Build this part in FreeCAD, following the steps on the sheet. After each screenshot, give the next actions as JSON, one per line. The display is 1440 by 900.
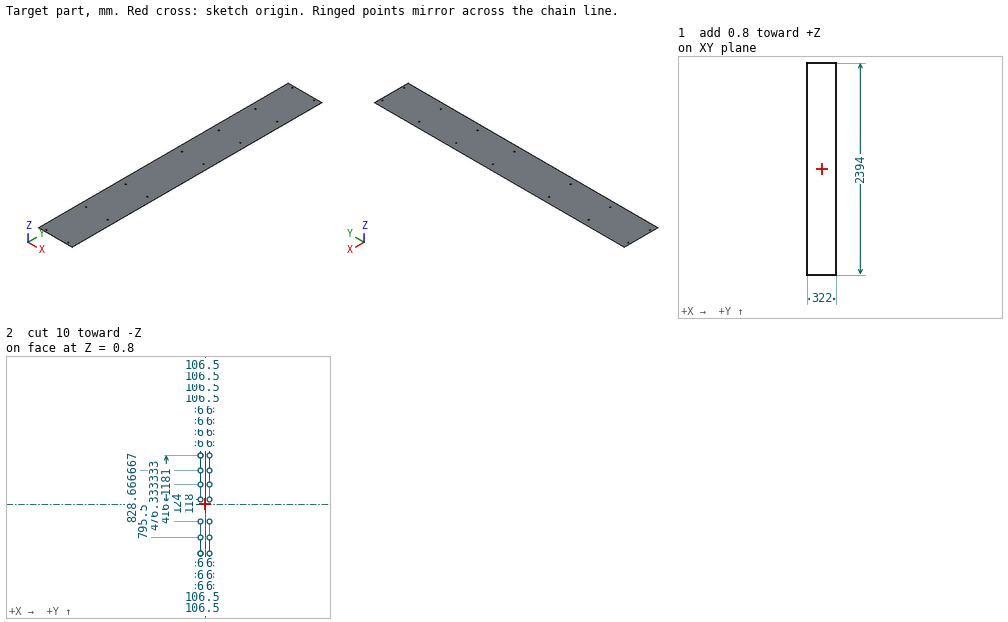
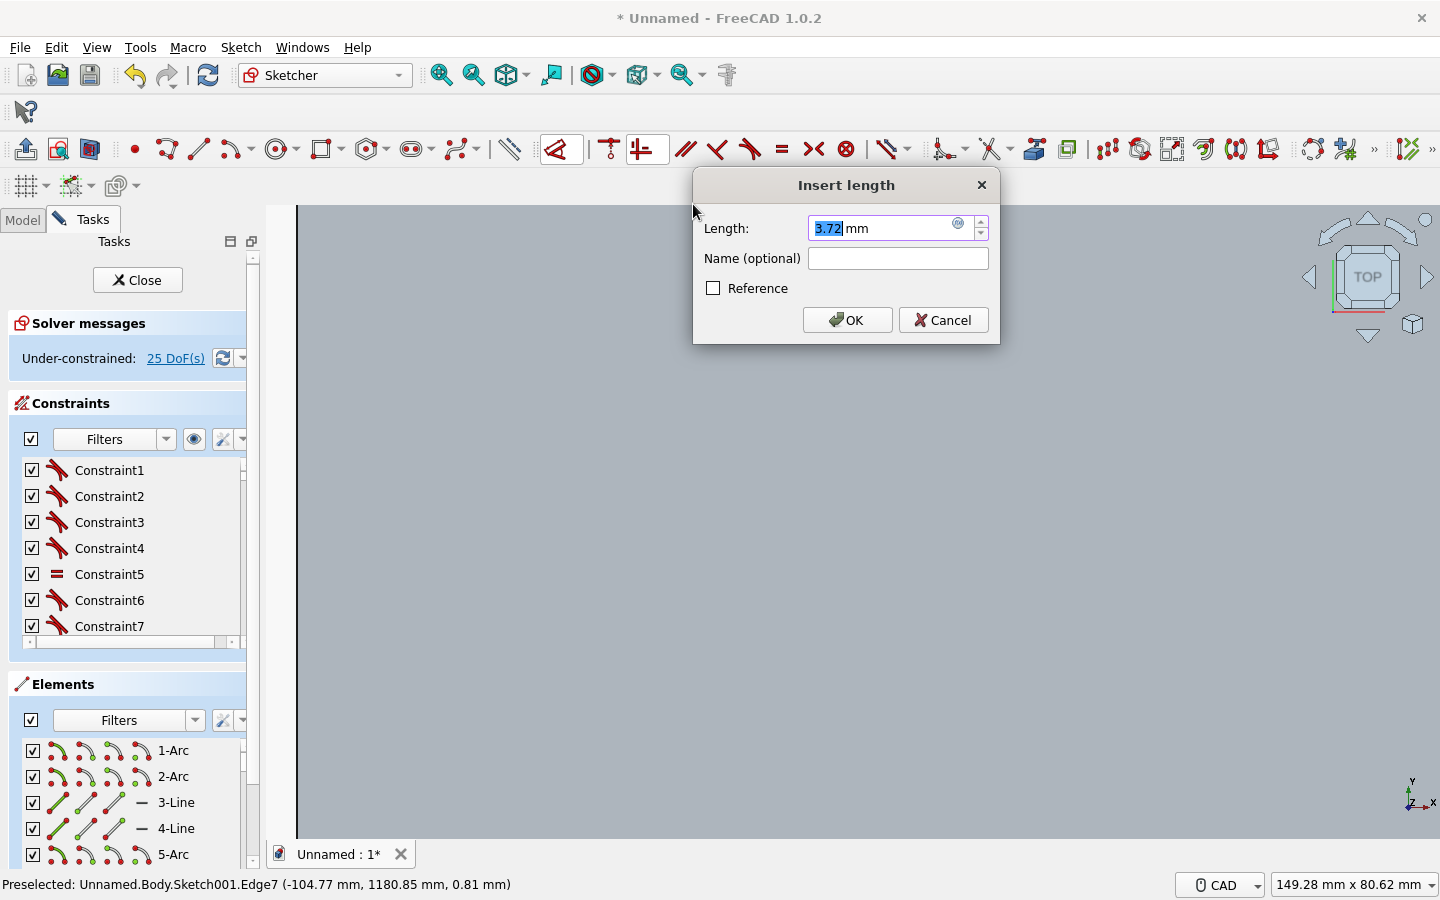
{"action": "type", "text": "6"}
{"action": "key", "text": "Return"}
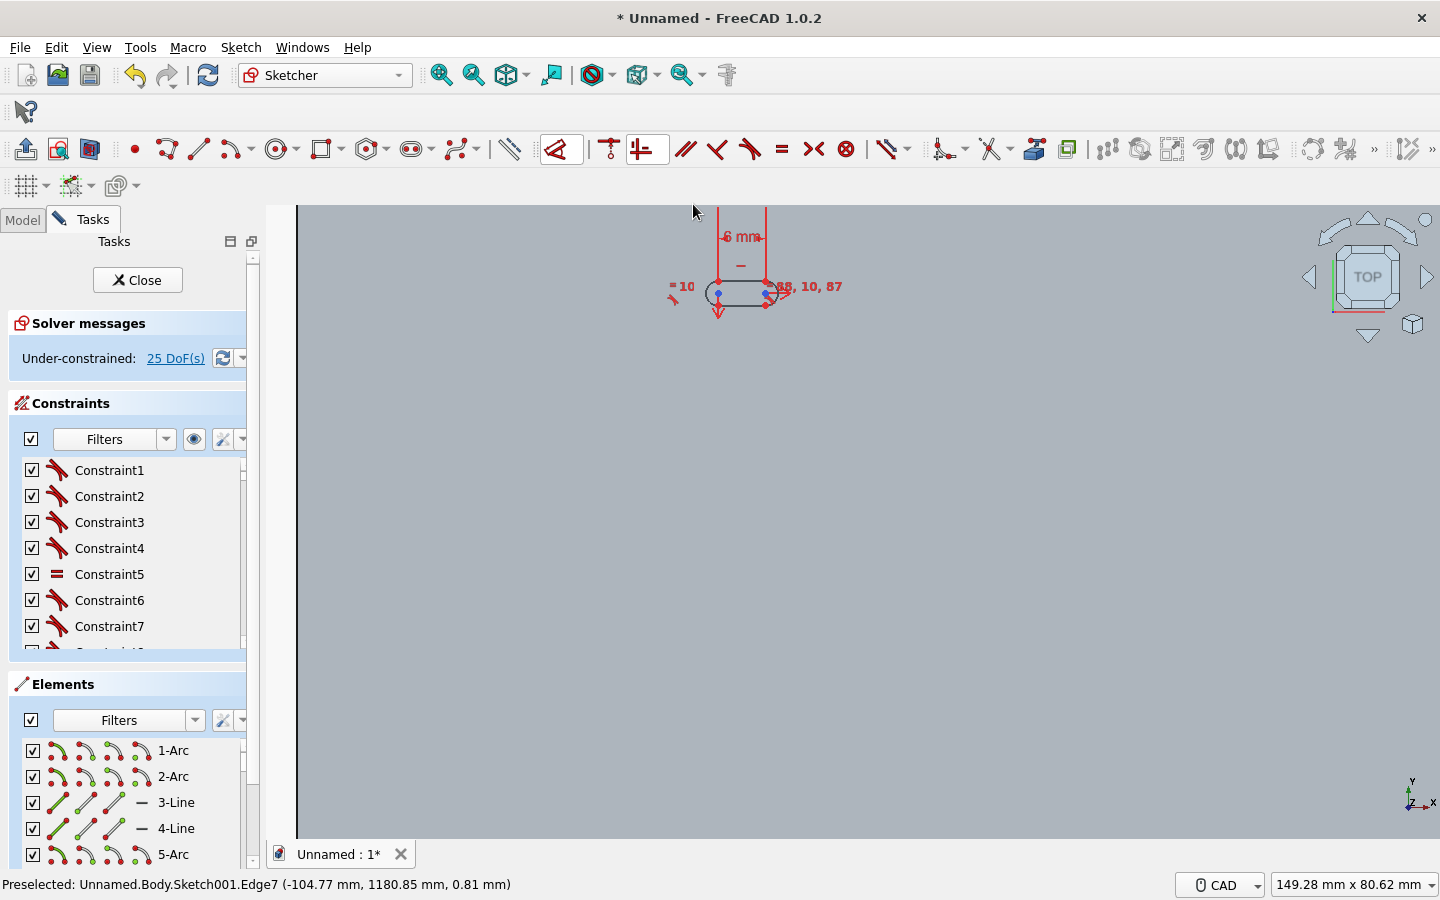
{"action": "scroll", "coordinate": [763, 268], "scroll_direction": "down", "scroll_amount": 18}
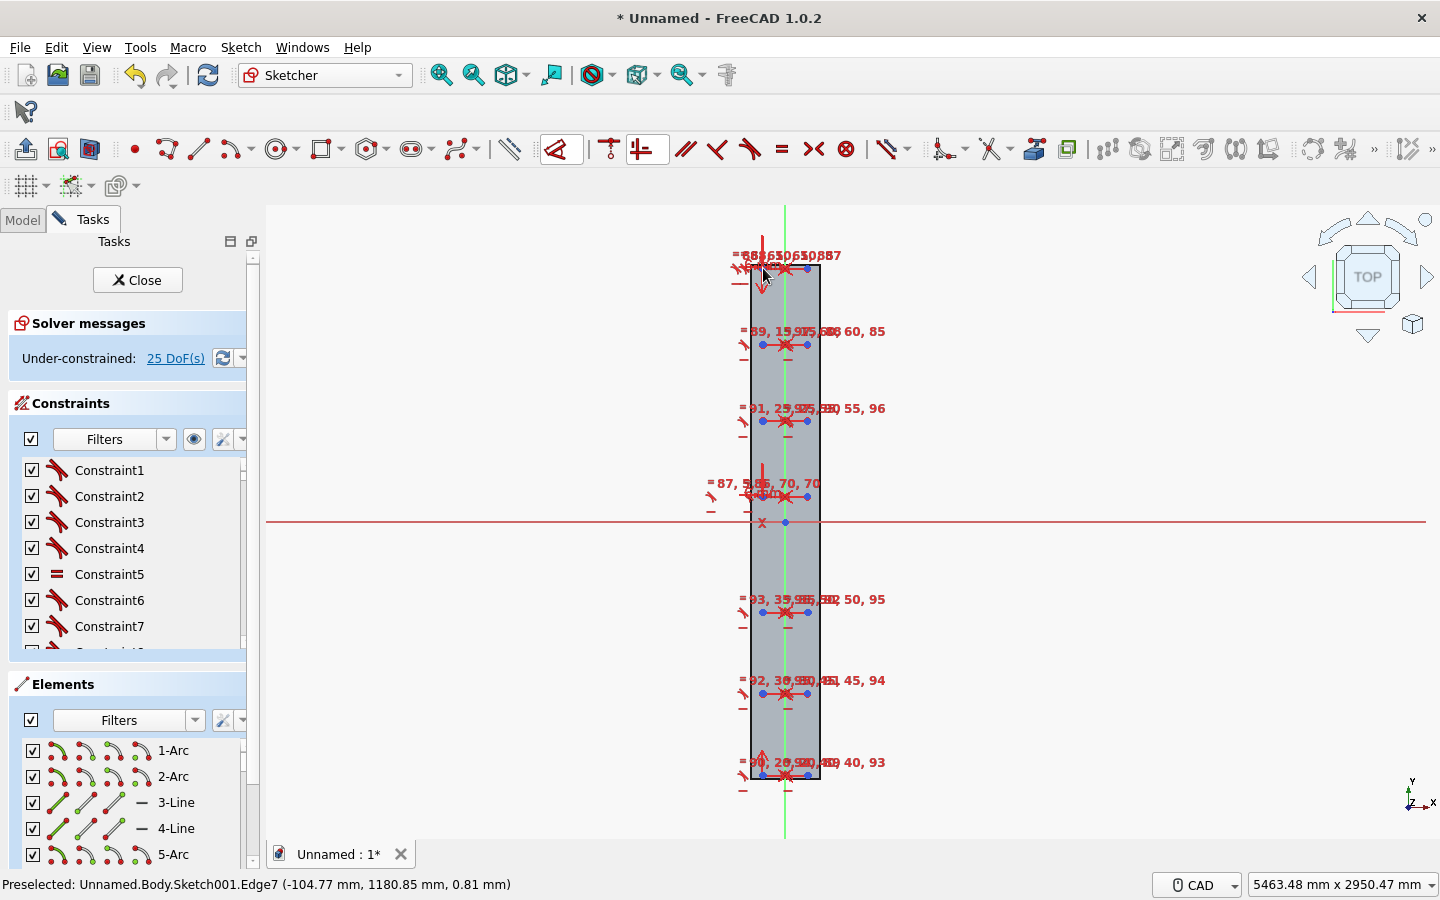
{"action": "scroll", "coordinate": [763, 345], "scroll_direction": "up", "scroll_amount": 18}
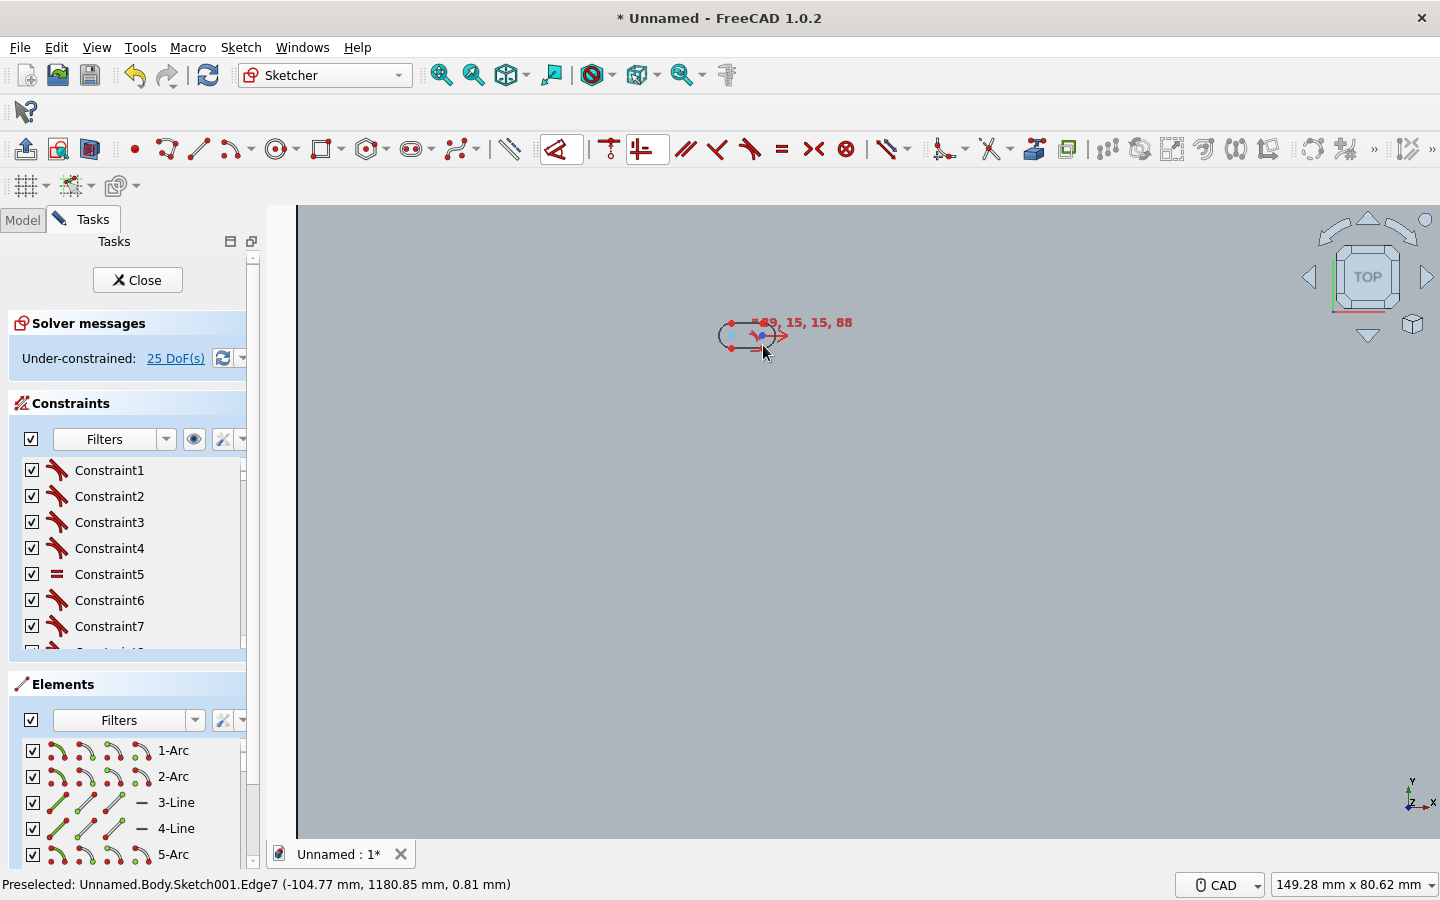
{"action": "left_click", "coordinate": [741, 323]}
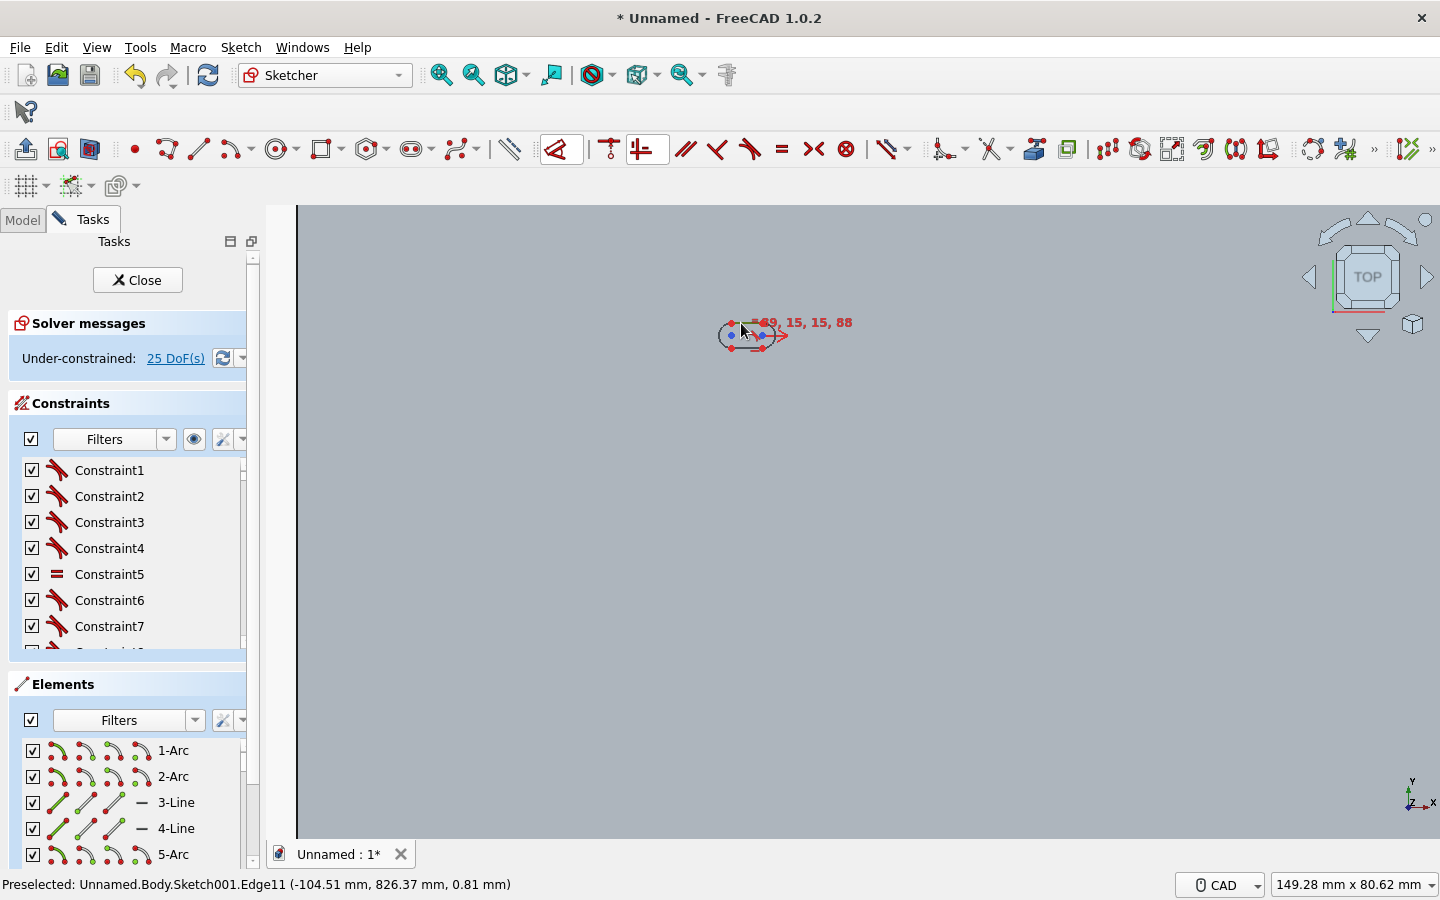
{"action": "key", "text": "l"}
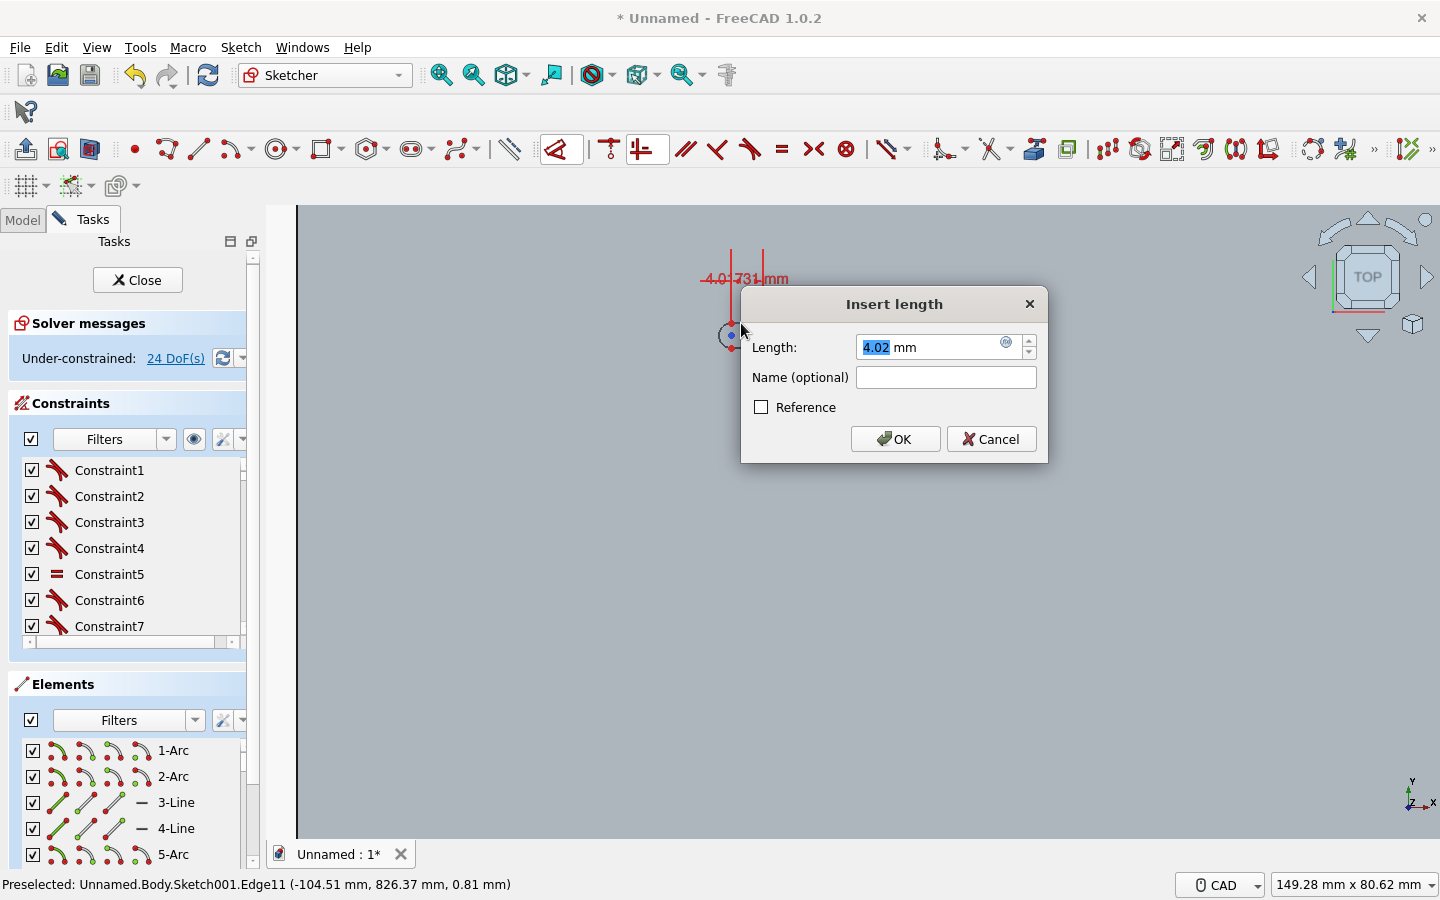
{"action": "type", "text": "6"}
{"action": "key", "text": "Return"}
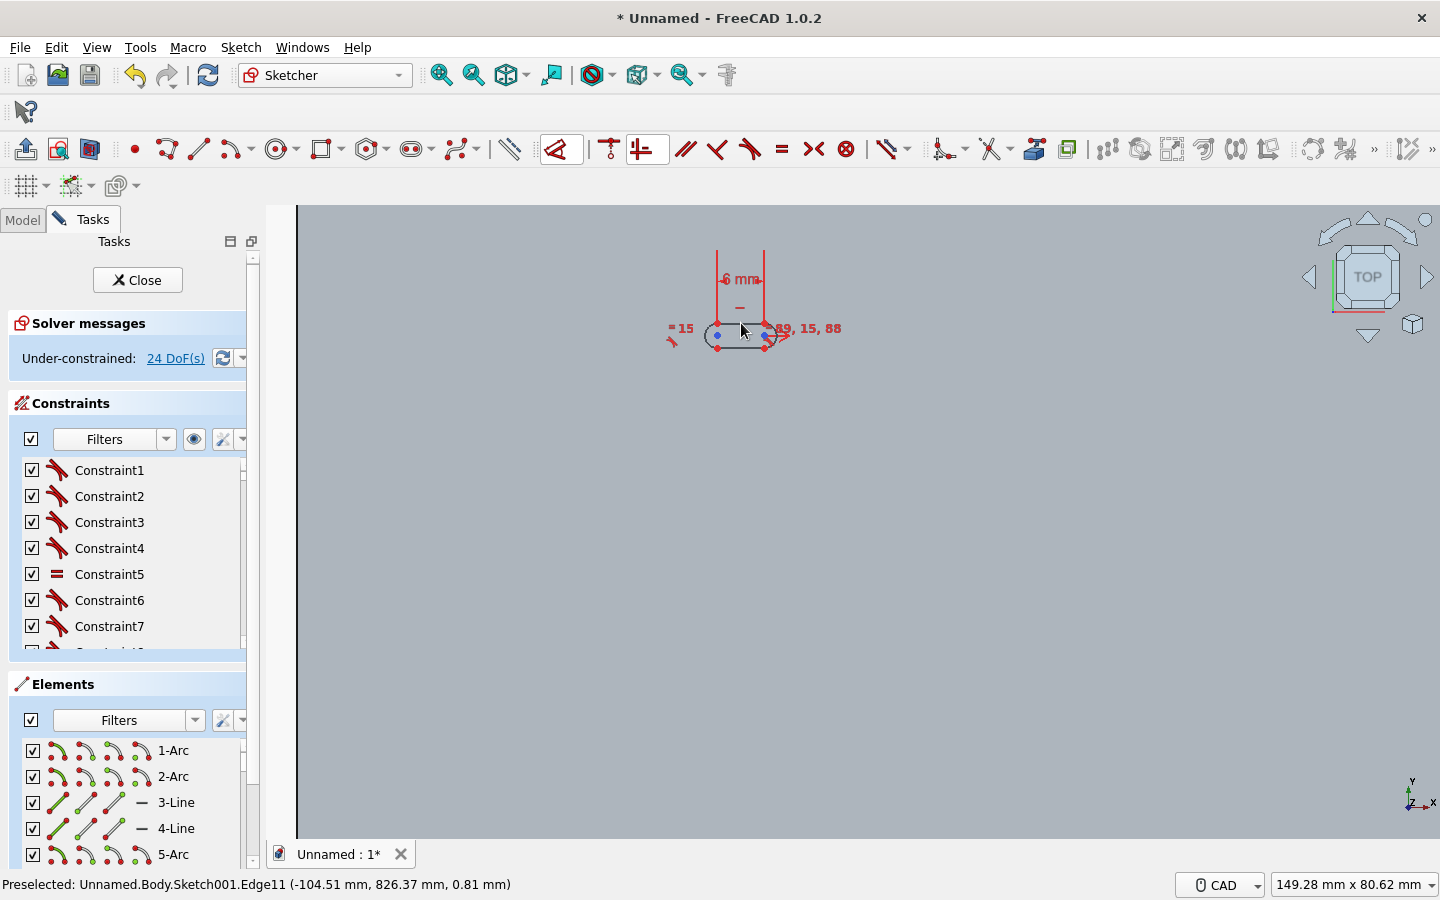
{"action": "scroll", "coordinate": [763, 345], "scroll_direction": "down", "scroll_amount": 18}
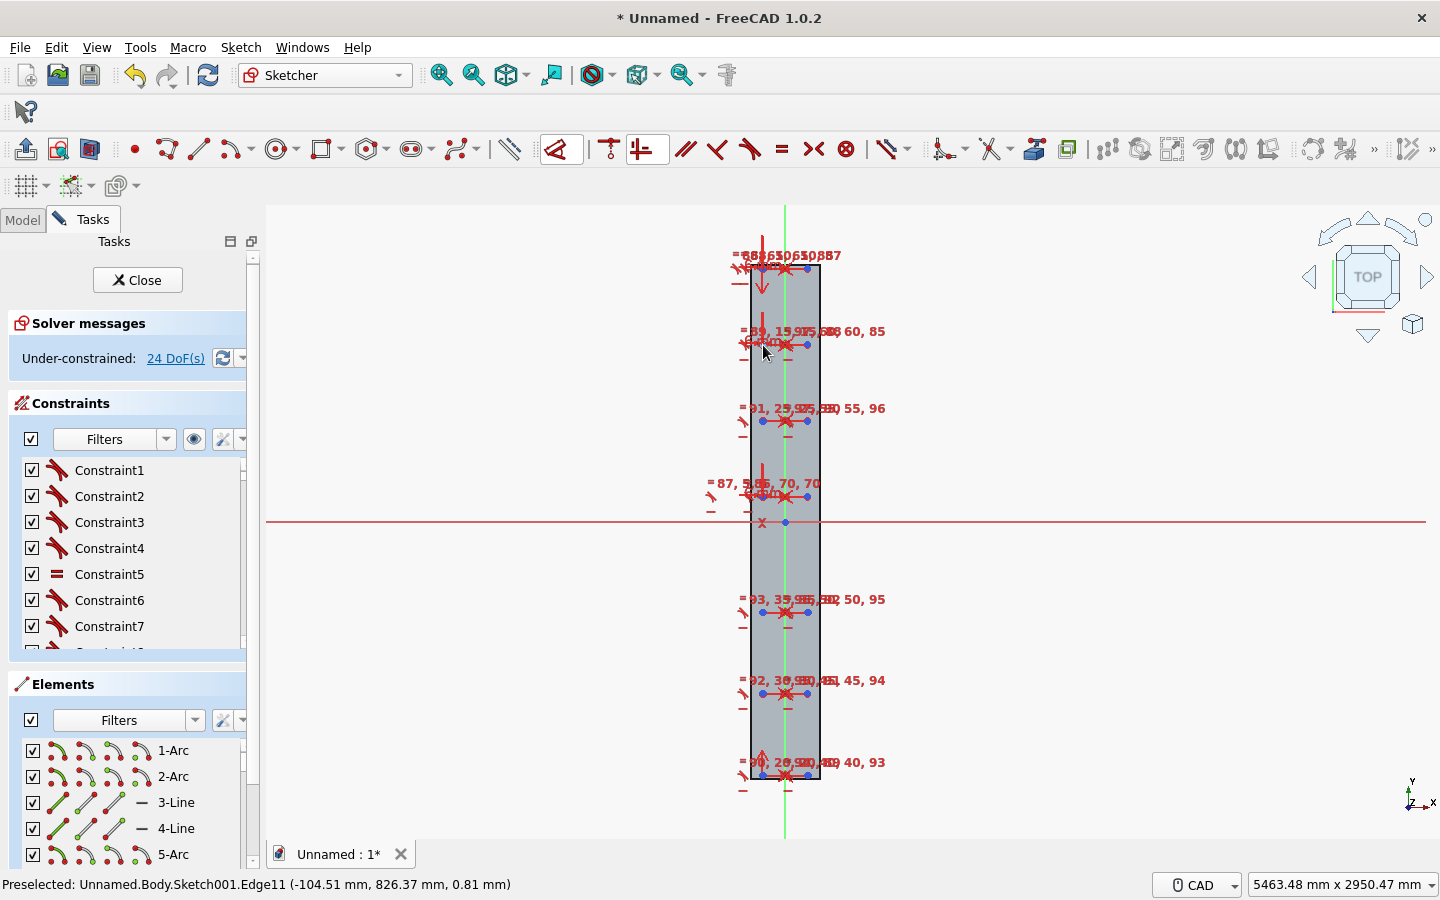
{"action": "scroll", "coordinate": [763, 775], "scroll_direction": "up", "scroll_amount": 18}